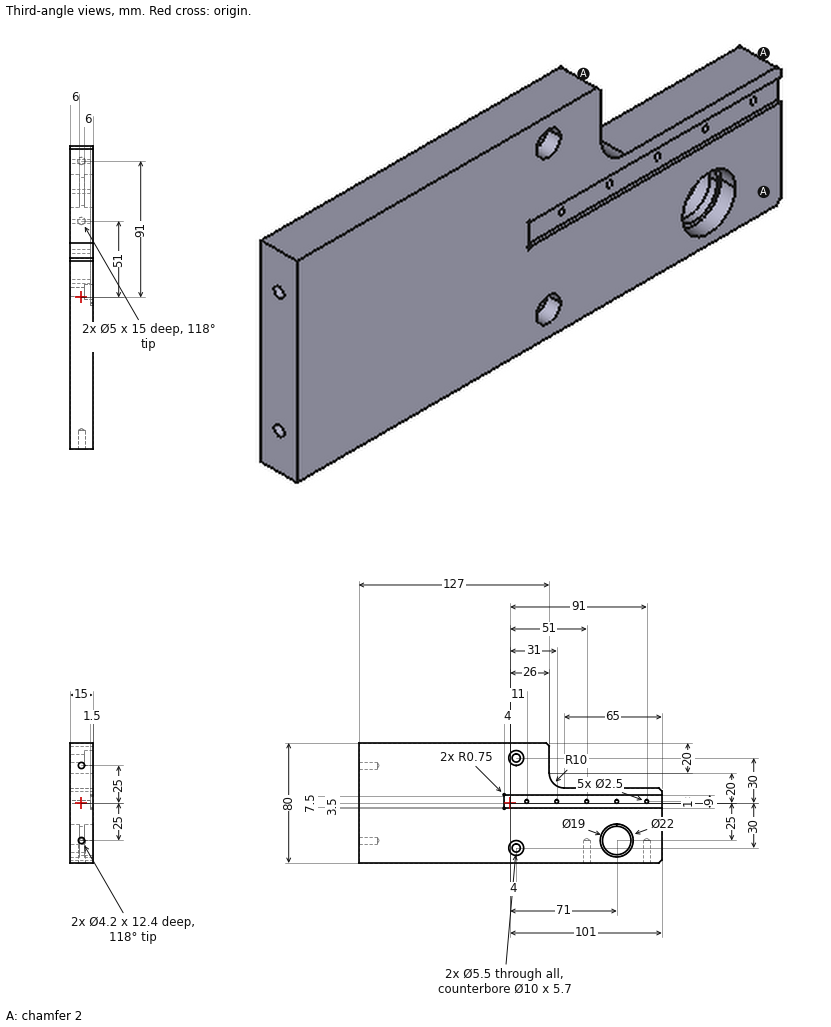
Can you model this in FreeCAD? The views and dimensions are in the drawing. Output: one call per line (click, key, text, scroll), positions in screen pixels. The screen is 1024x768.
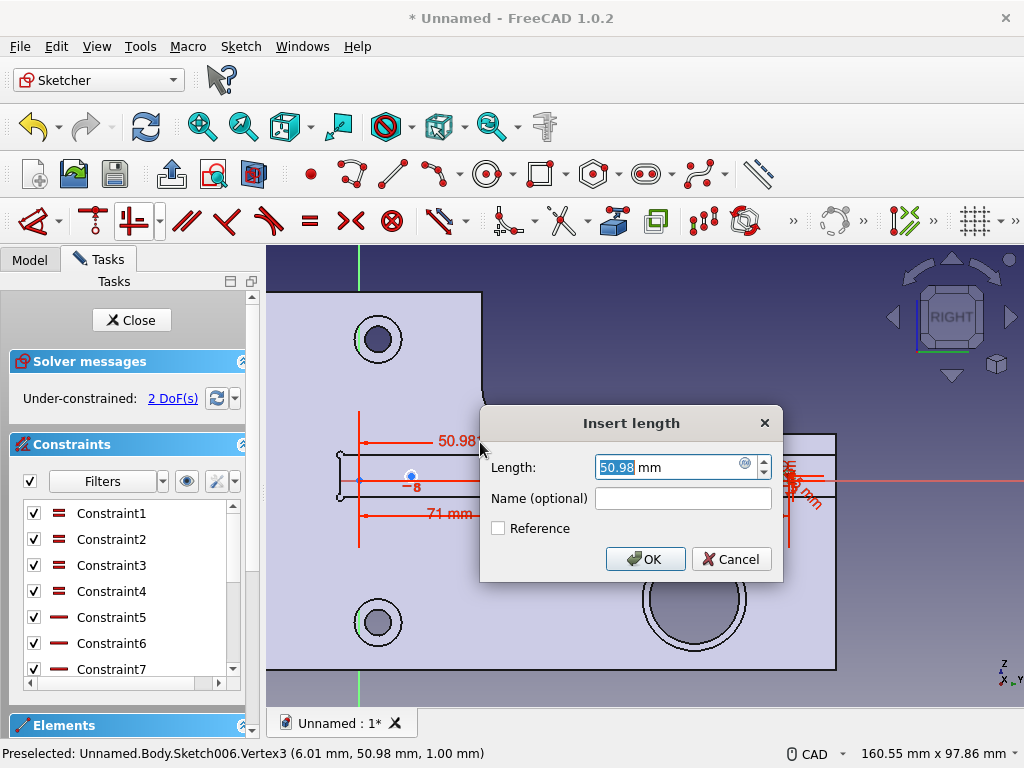
text(51)
key(Return)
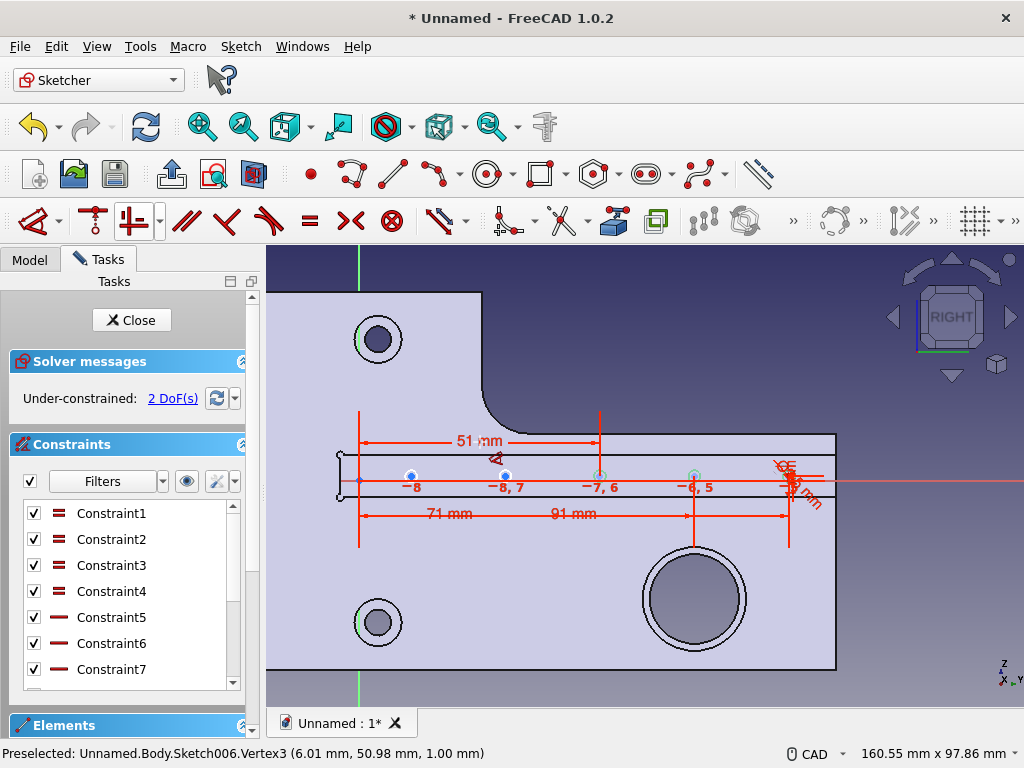
click(506, 476)
click(399, 442)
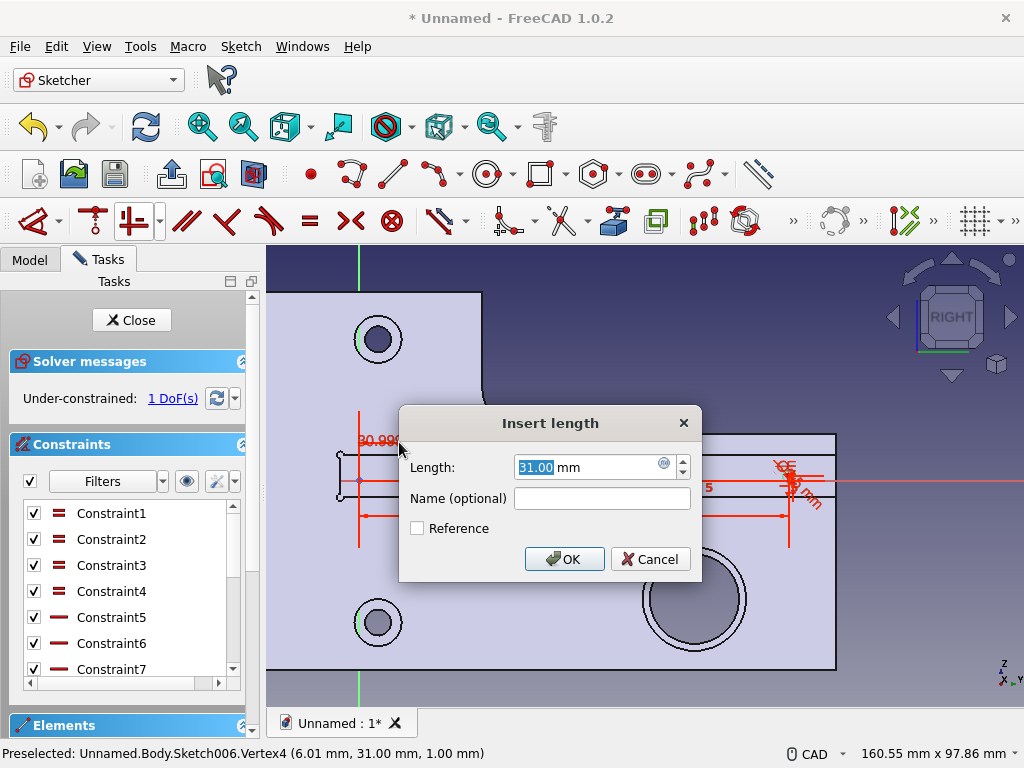
text(31)
key(Return)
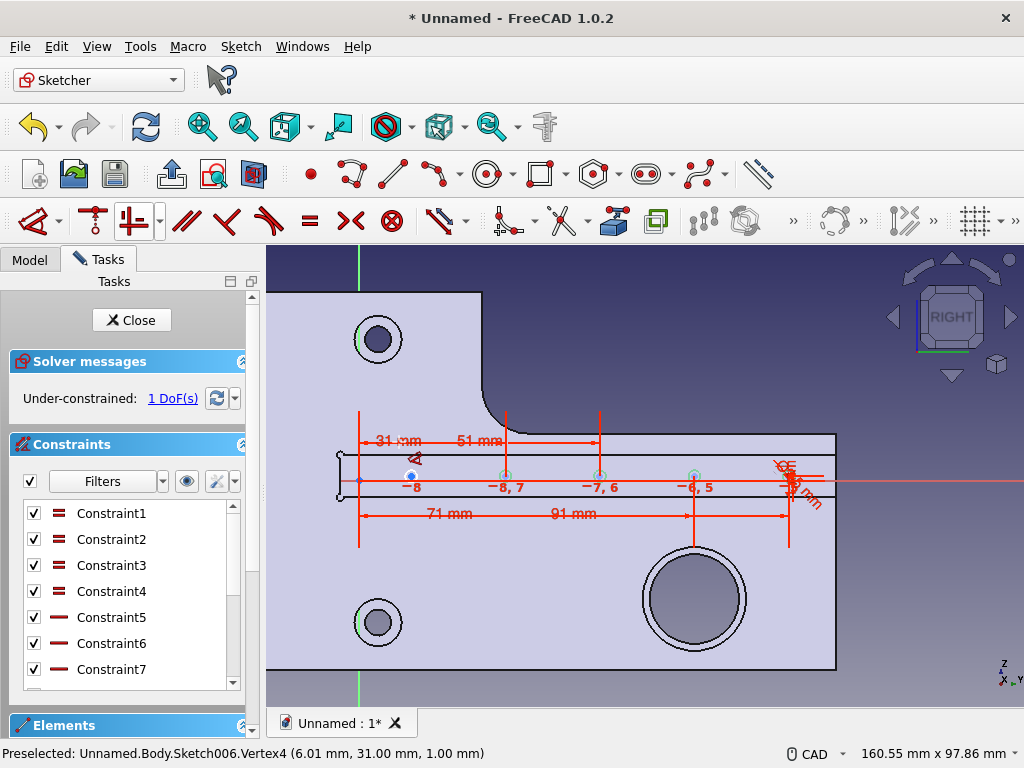
click(411, 476)
click(373, 515)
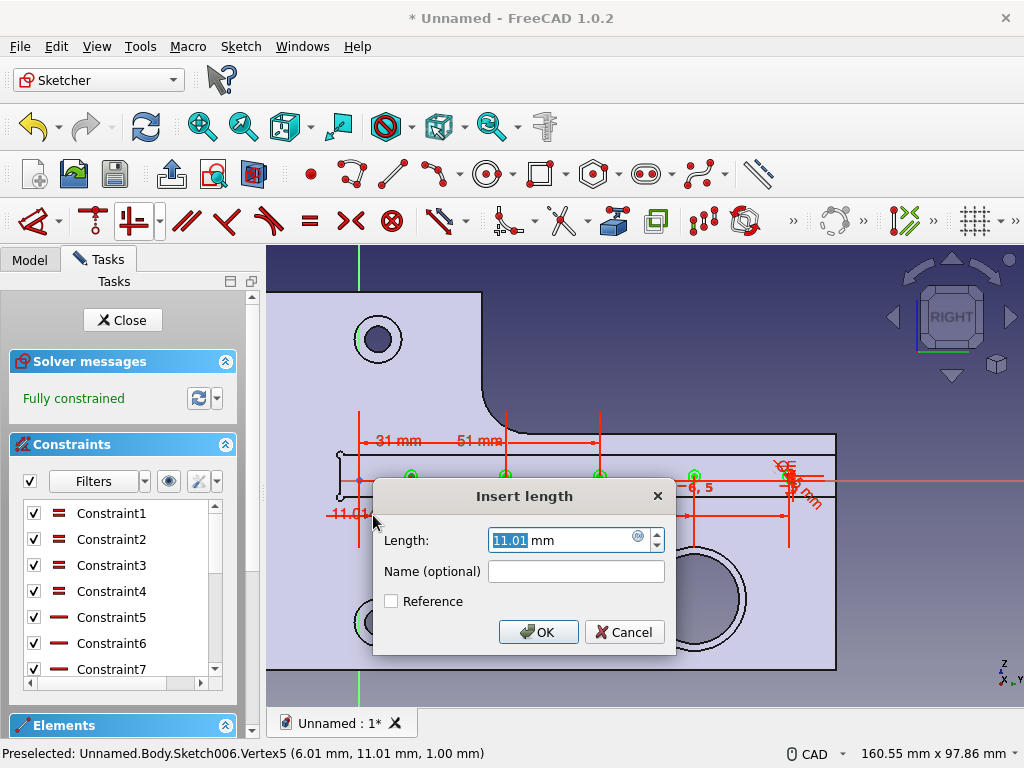
text(11)
key(Return)
key(Escape)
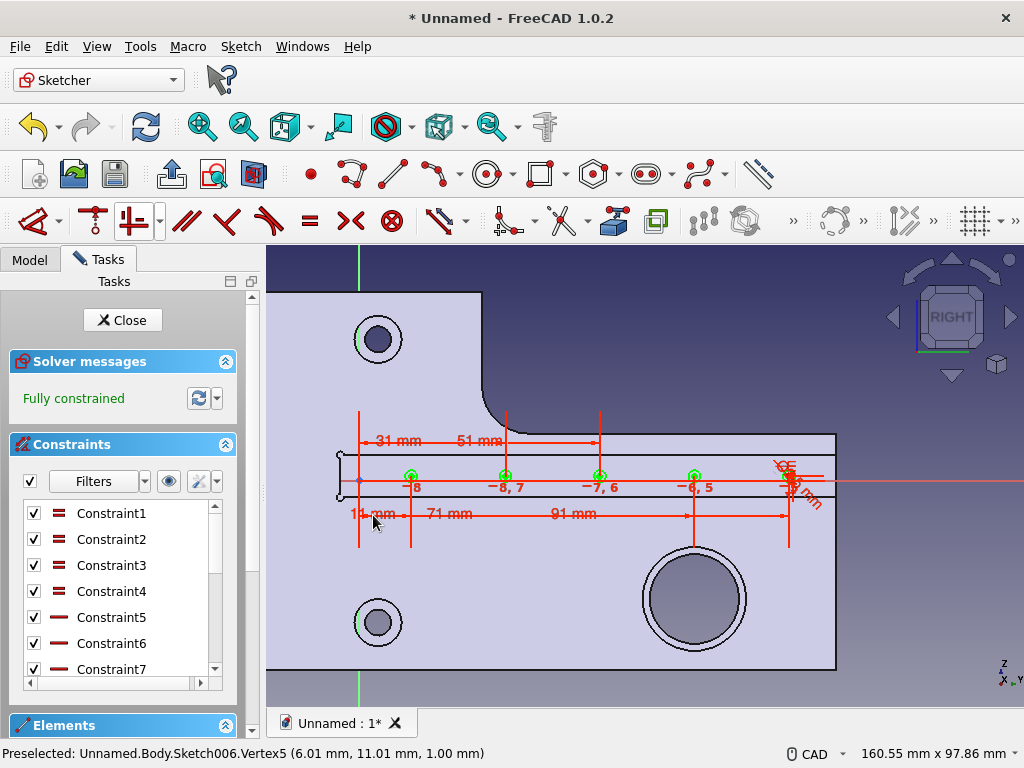
click(123, 320)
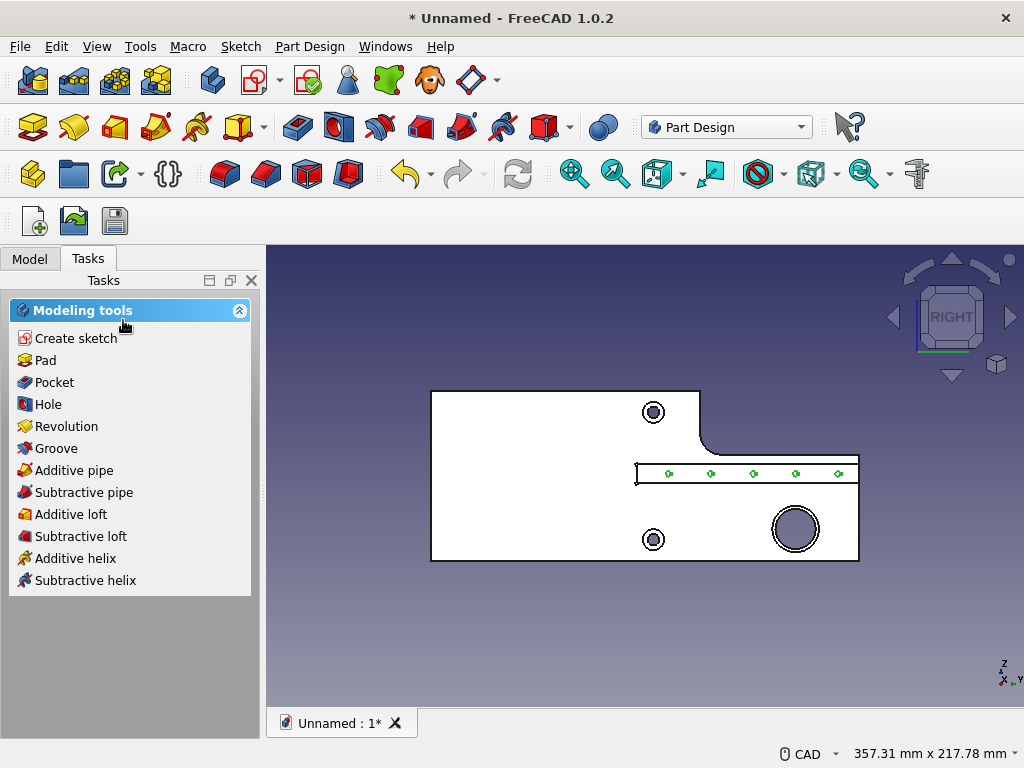
click(298, 128)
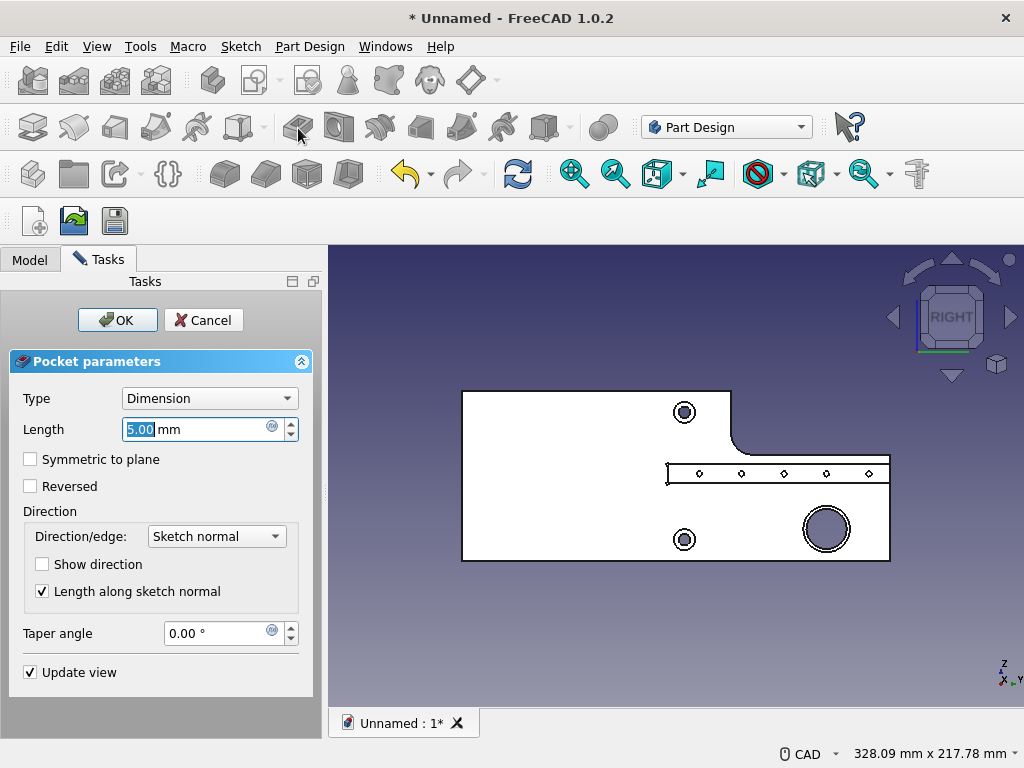
click(210, 398)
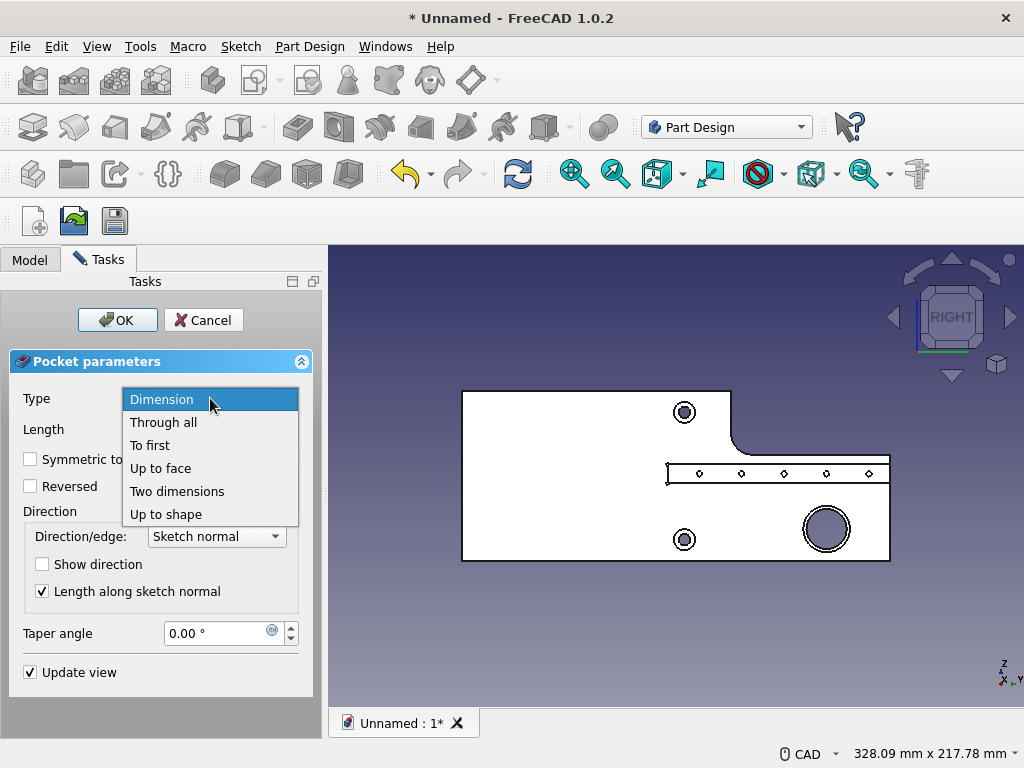
click(208, 422)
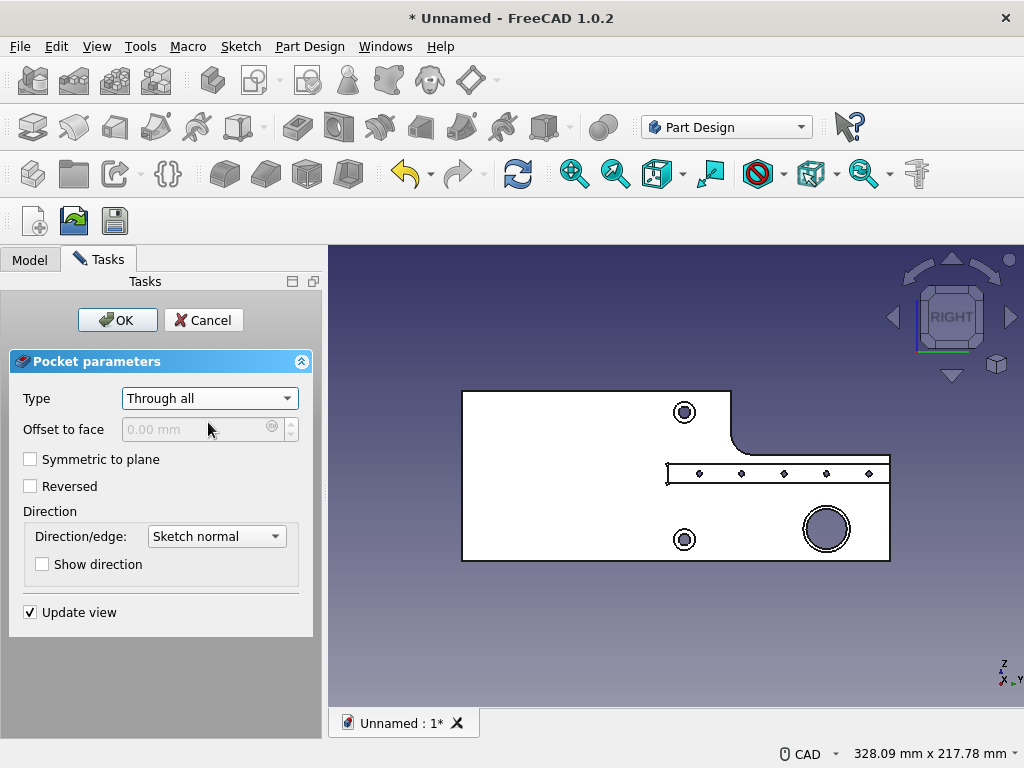
click(118, 320)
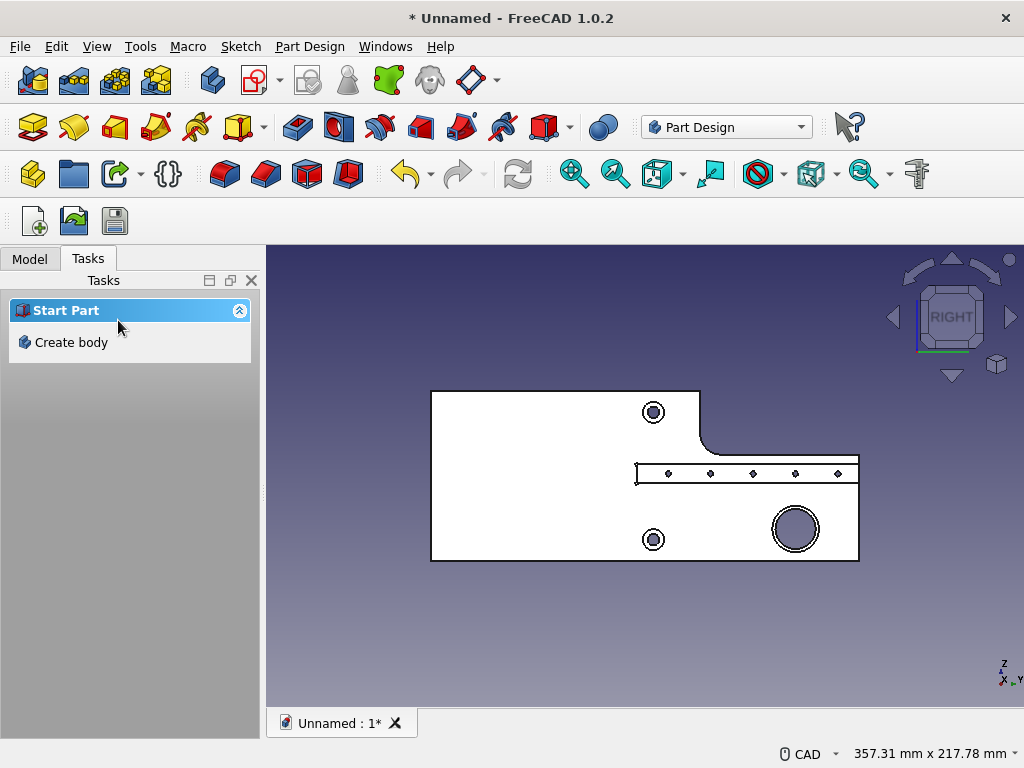
click(30, 258)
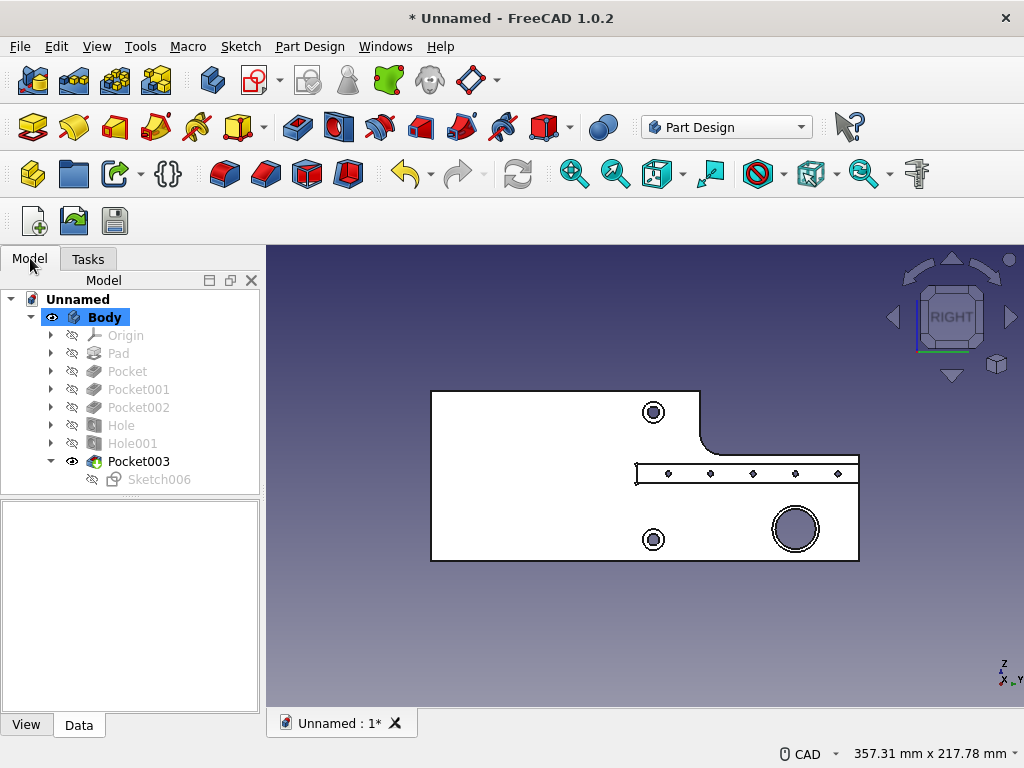
click(51, 335)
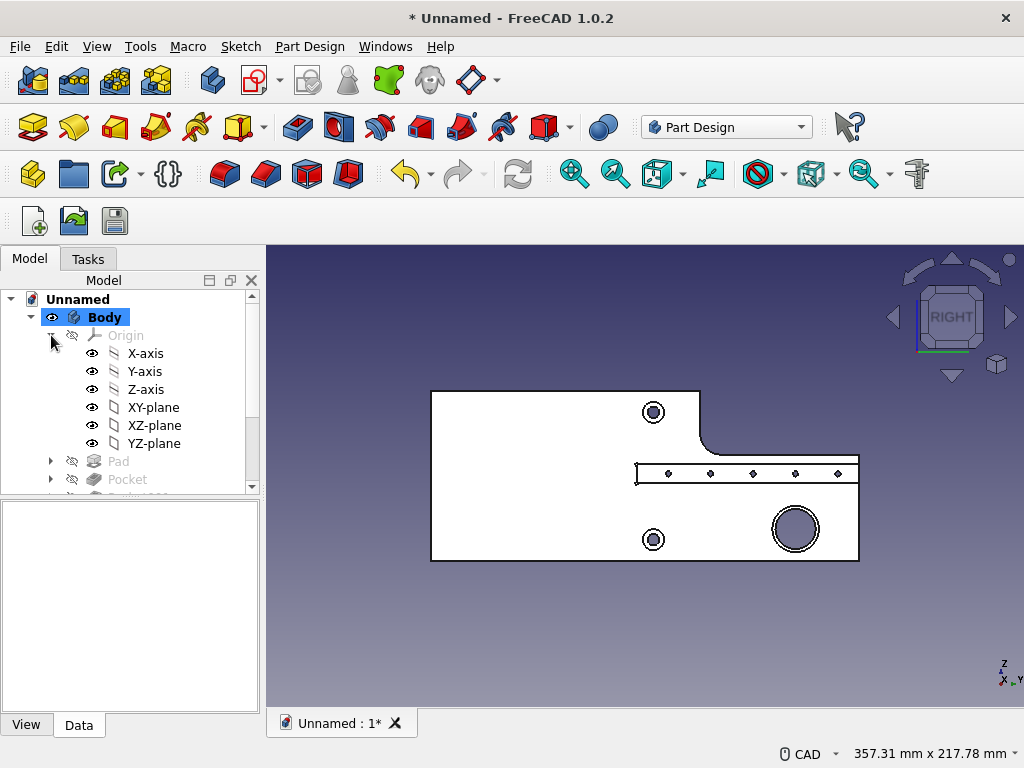
click(137, 443)